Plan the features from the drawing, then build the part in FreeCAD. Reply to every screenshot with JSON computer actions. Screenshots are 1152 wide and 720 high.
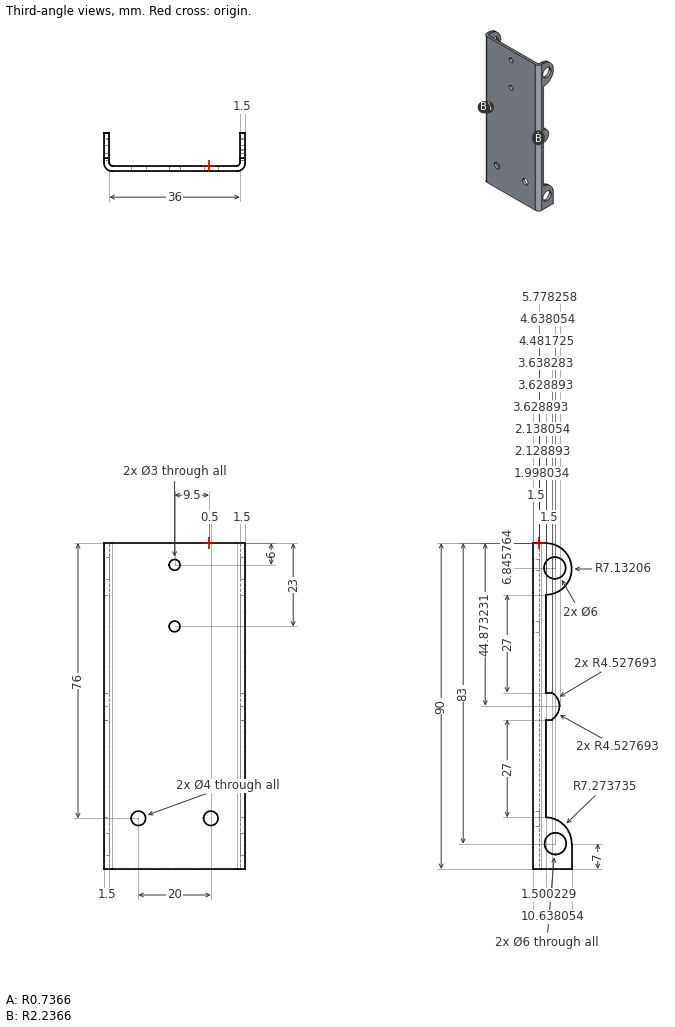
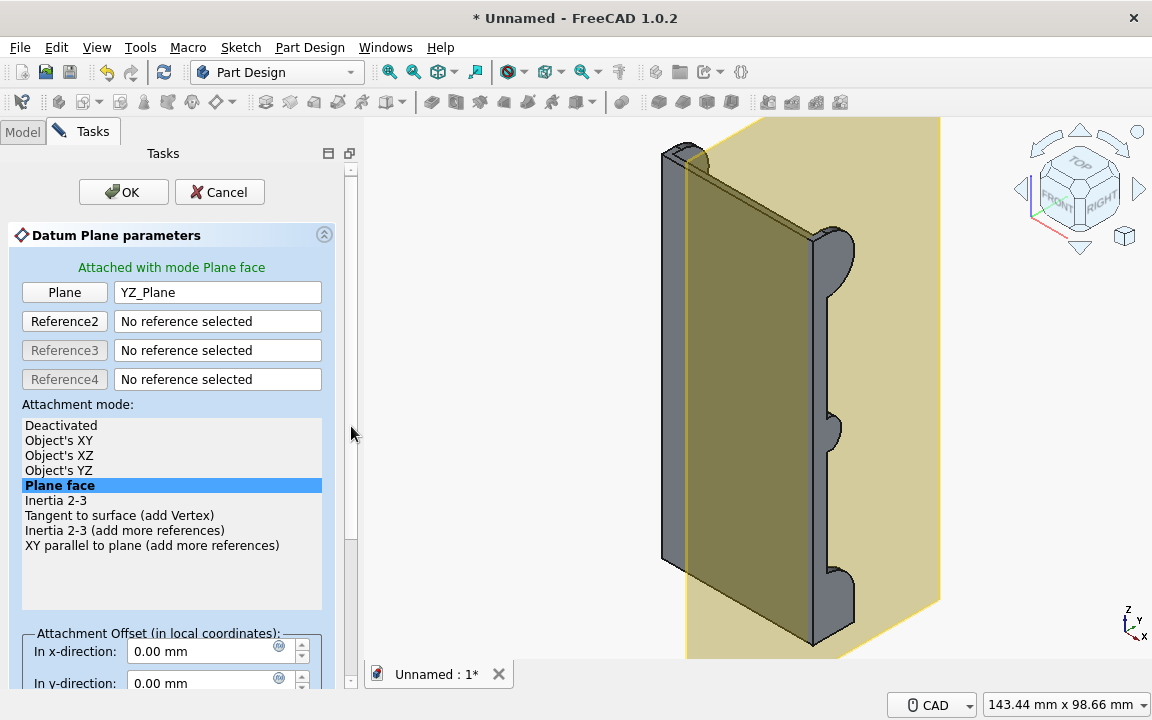
{"action": "left_click", "coordinate": [124, 192]}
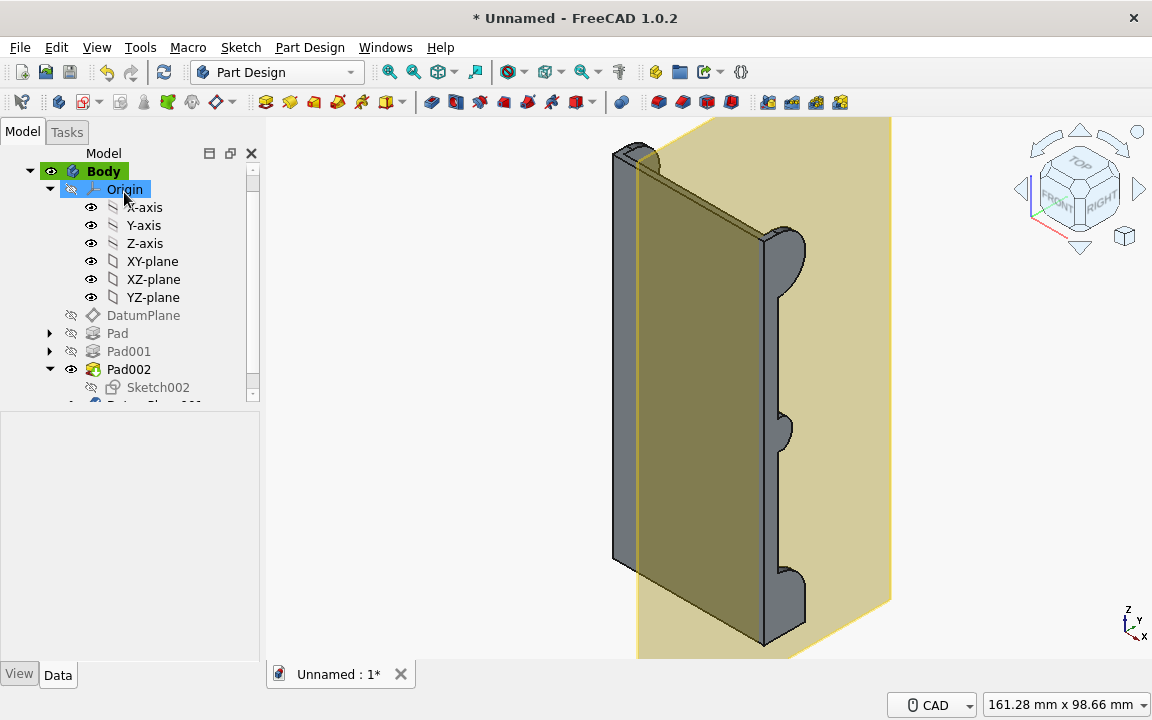
{"action": "scroll", "coordinate": [120, 275], "scroll_direction": "down", "scroll_amount": 3}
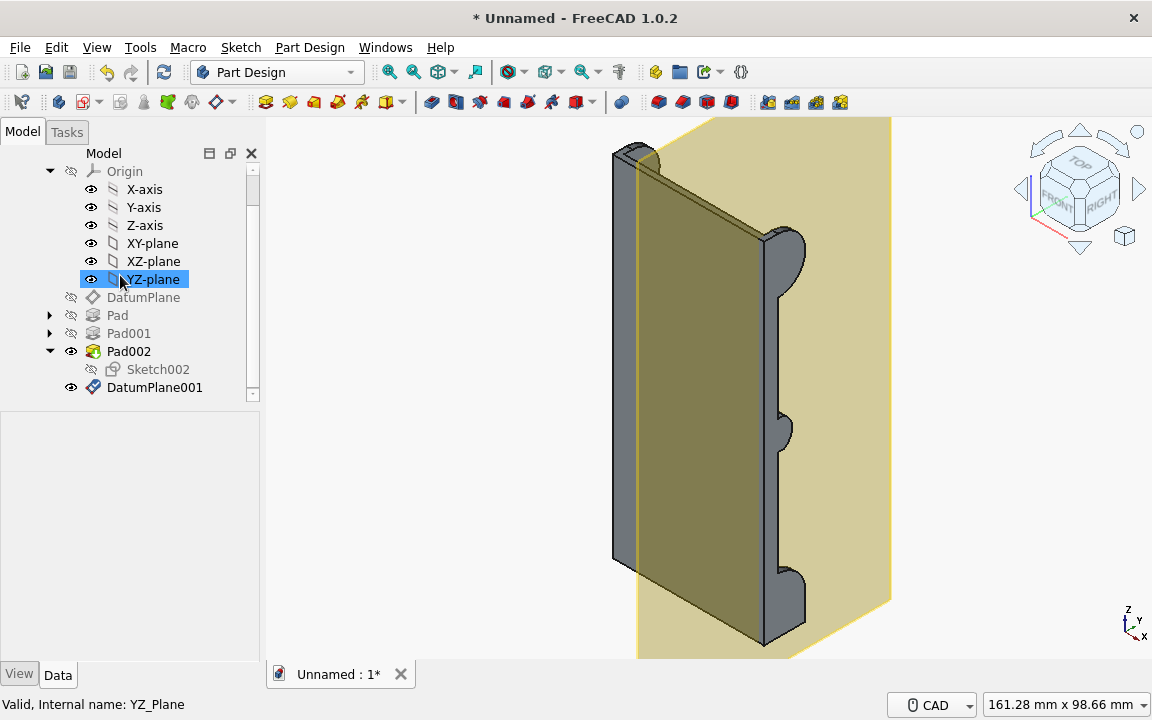
{"action": "left_click", "coordinate": [116, 387]}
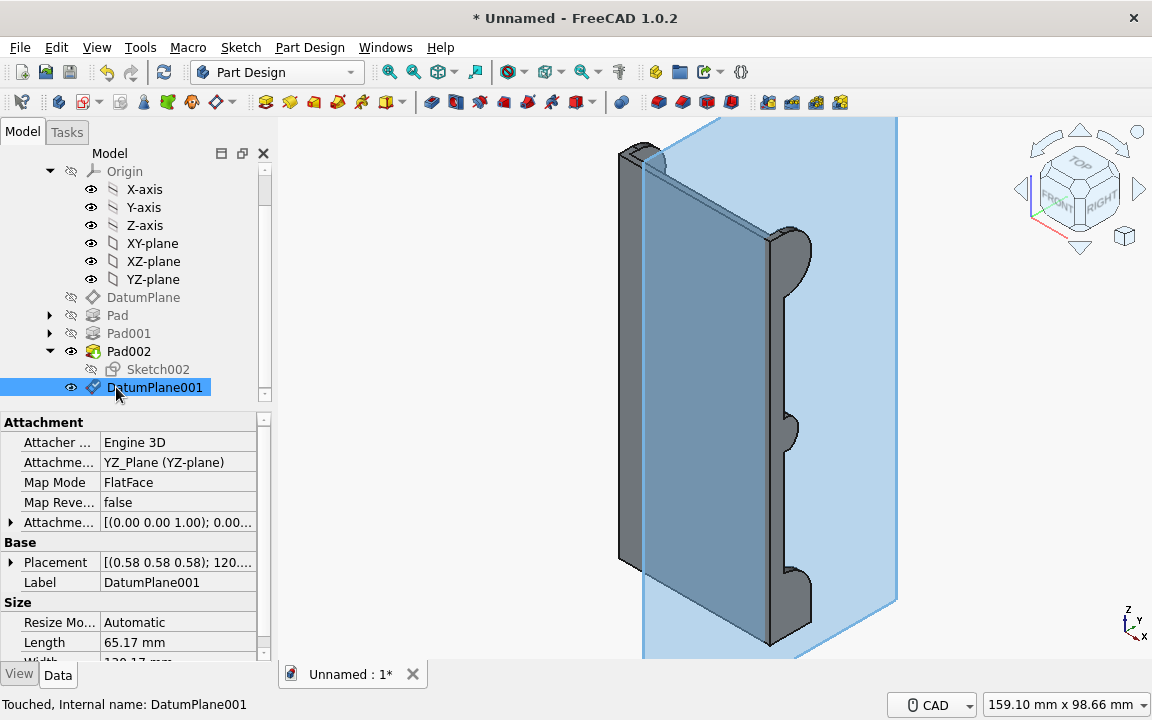
{"action": "left_click", "coordinate": [84, 102]}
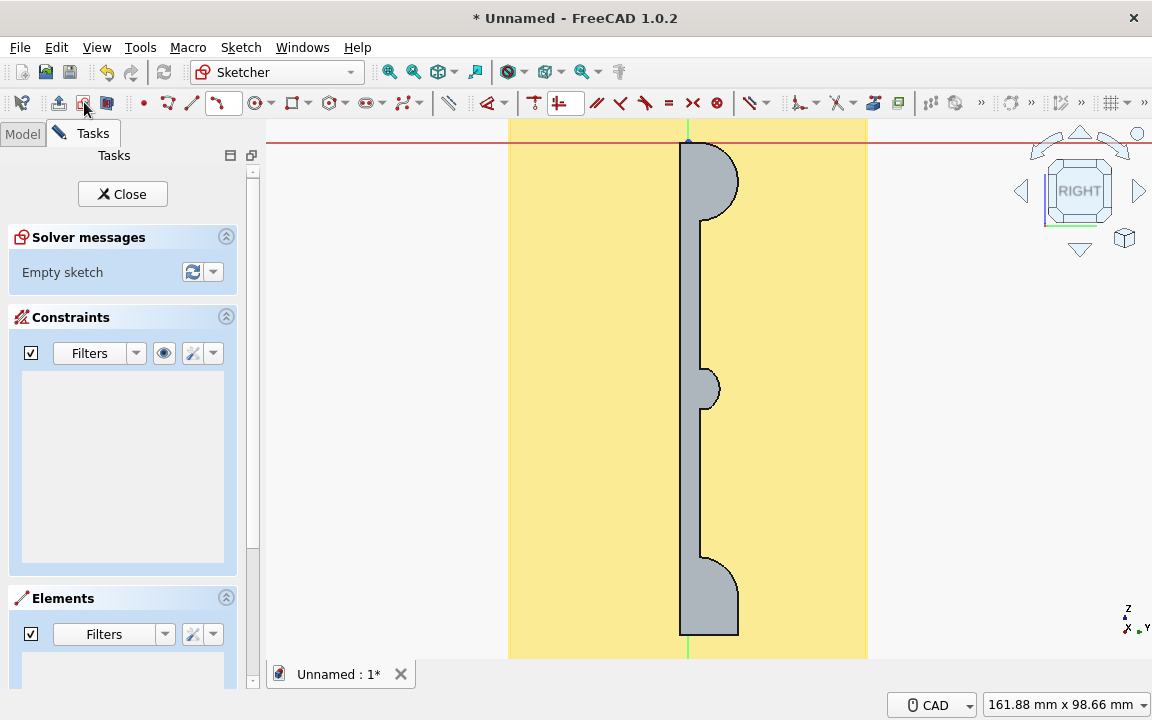
{"action": "key", "text": "q s"}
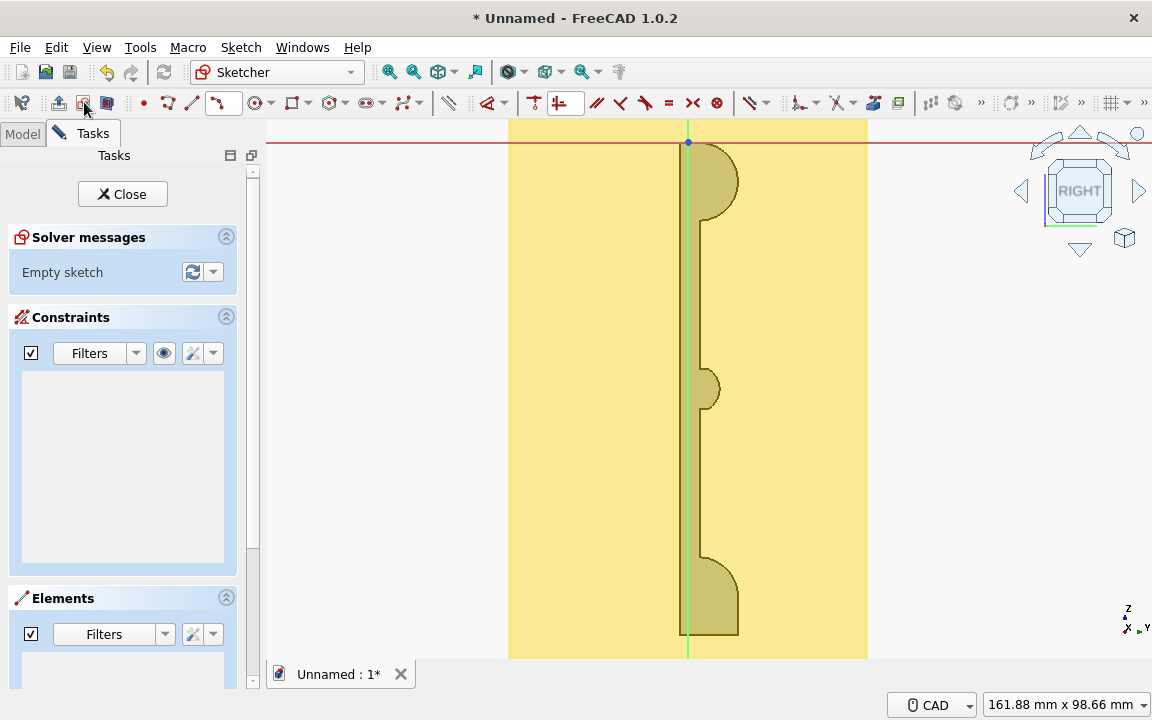
{"action": "scroll", "coordinate": [501, 411], "scroll_direction": "down", "scroll_amount": 2}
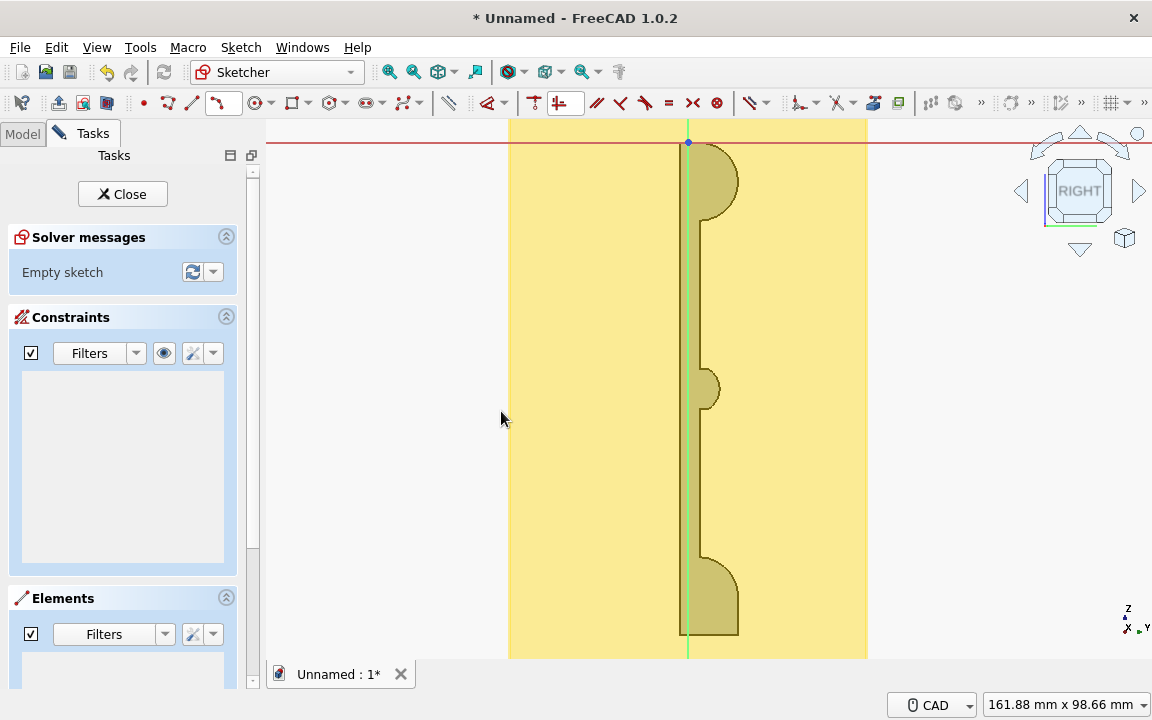
{"action": "left_click", "coordinate": [256, 104]}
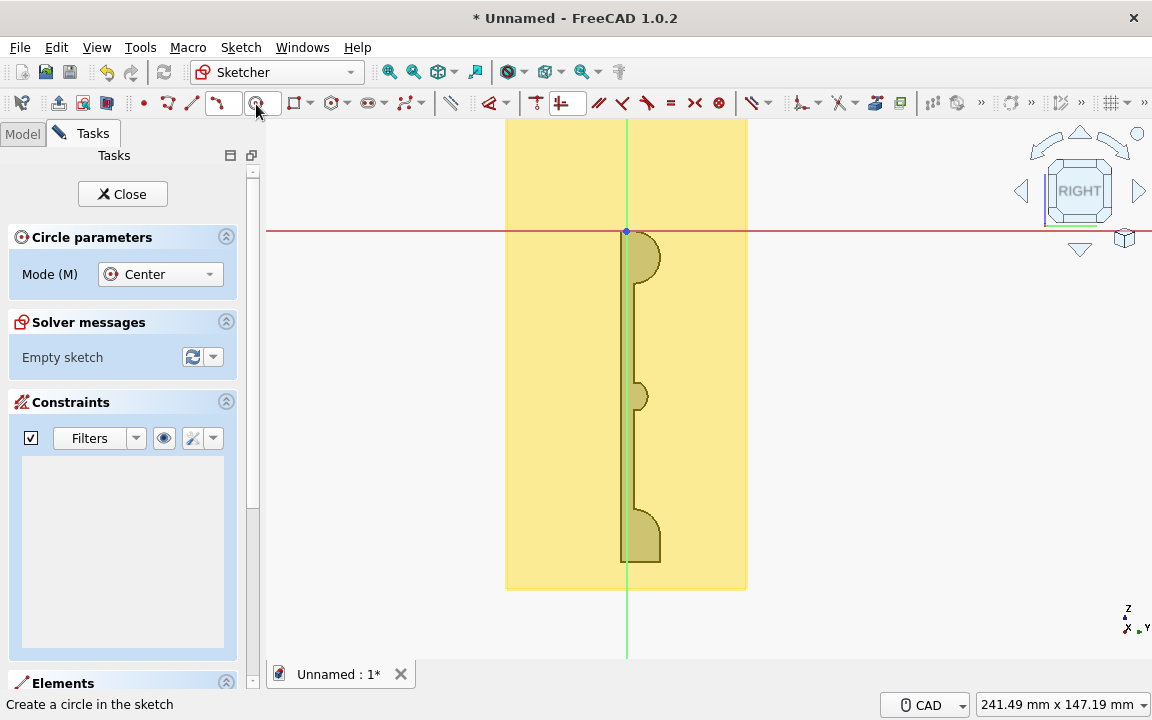
{"action": "scroll", "coordinate": [643, 256], "scroll_direction": "up", "scroll_amount": 4}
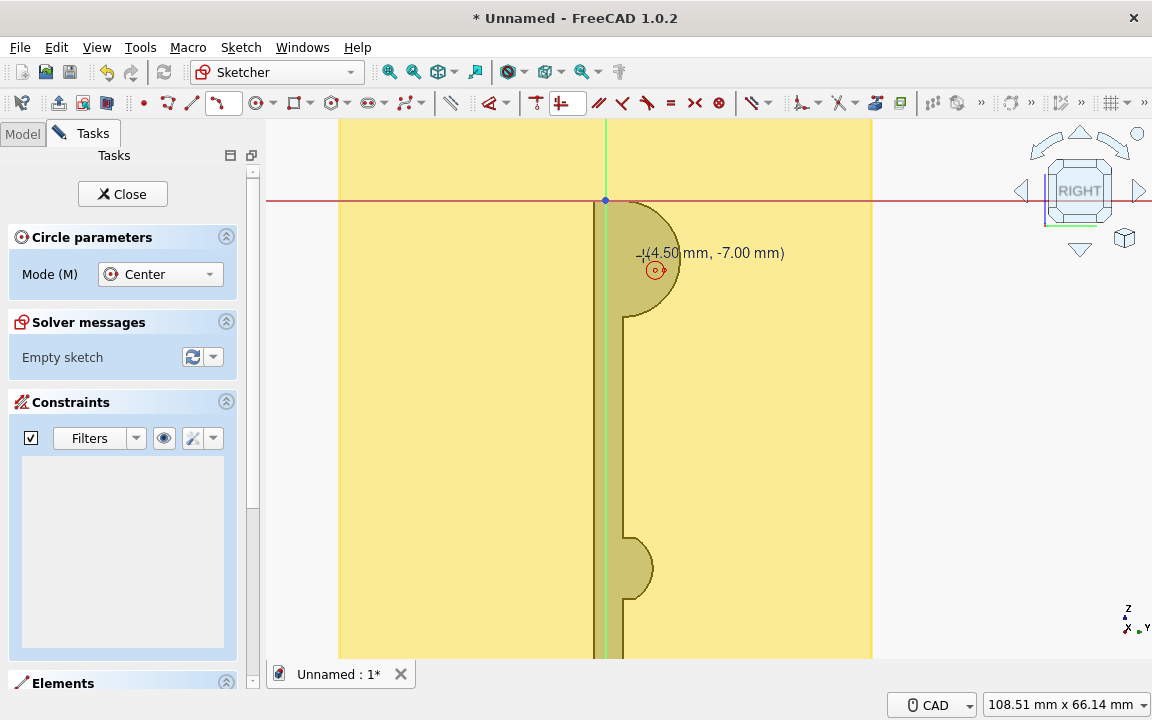
{"action": "left_click", "coordinate": [642, 257]}
{"action": "left_click", "coordinate": [660, 239]}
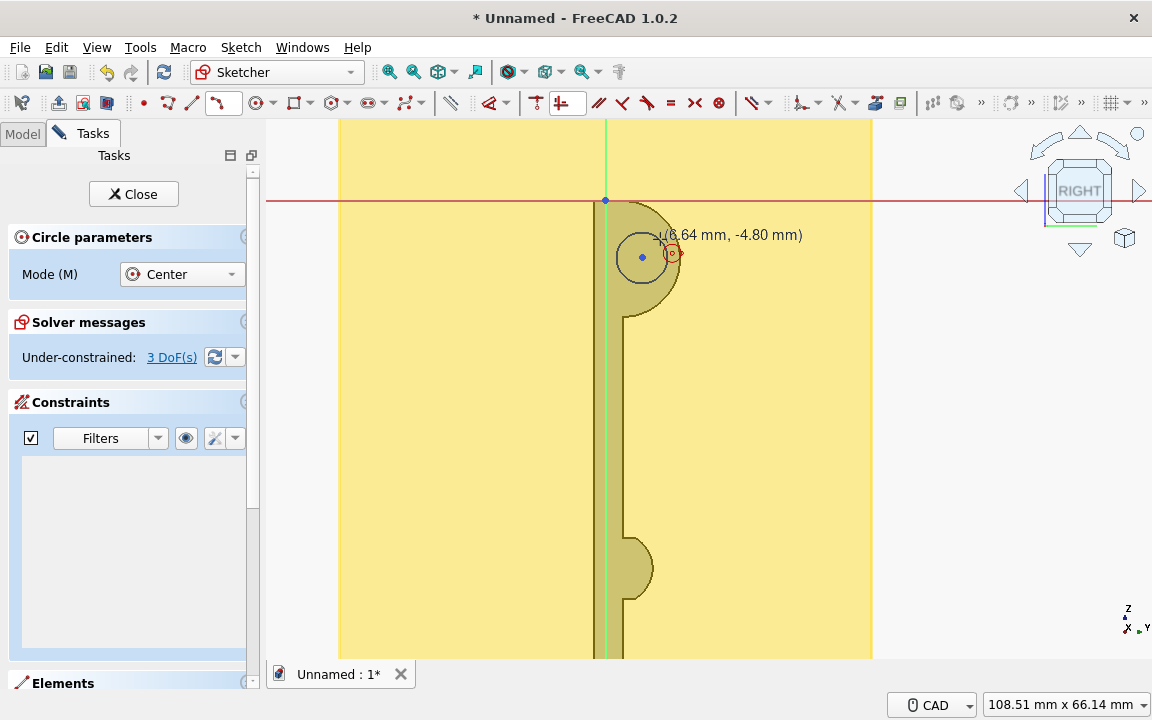
{"action": "scroll", "coordinate": [643, 256], "scroll_direction": "down", "scroll_amount": 4}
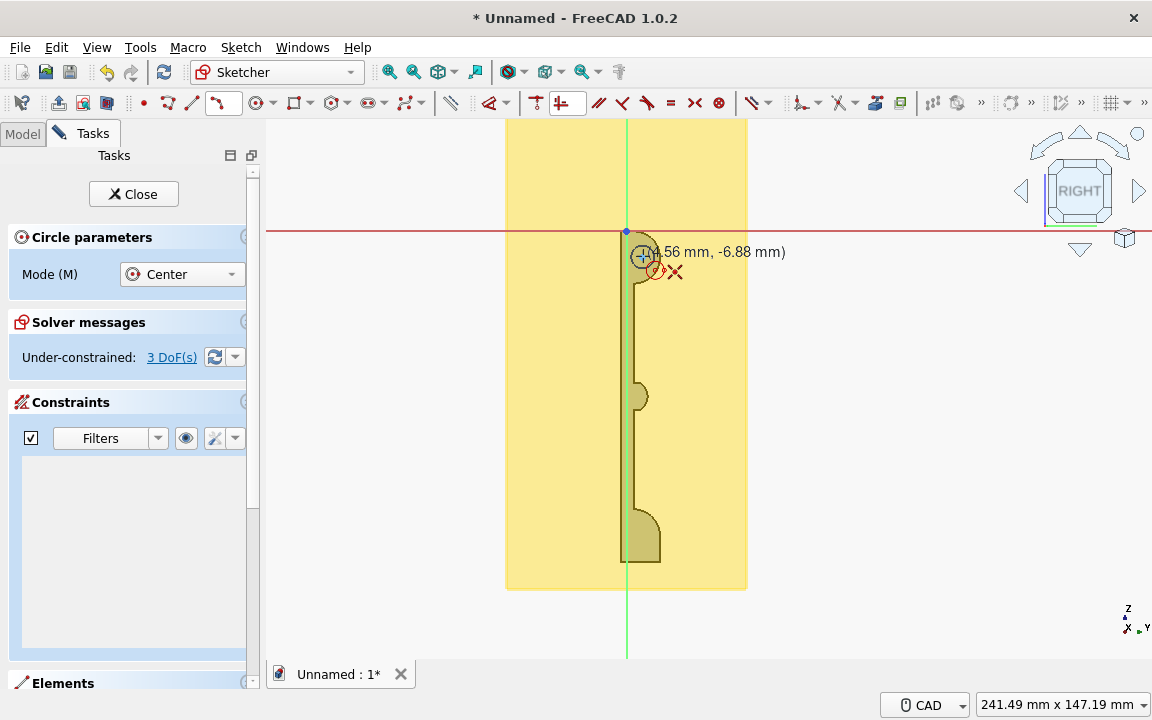
{"action": "scroll", "coordinate": [644, 536], "scroll_direction": "up", "scroll_amount": 4}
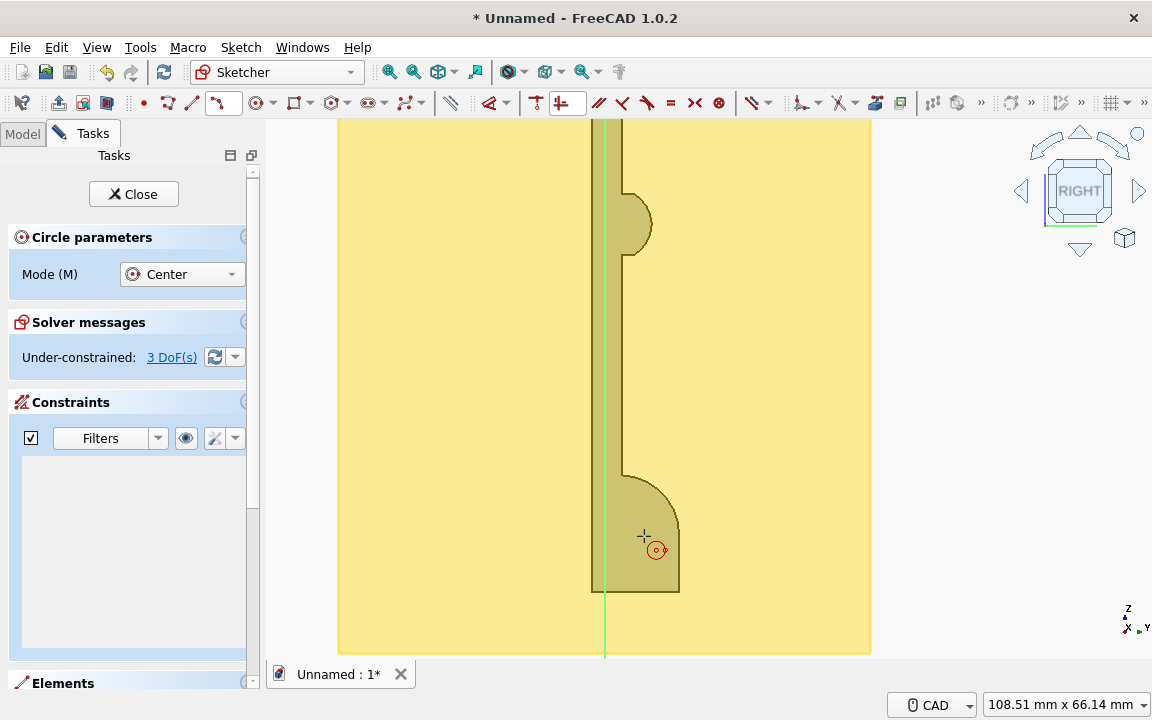
{"action": "left_click", "coordinate": [642, 535]}
{"action": "left_click", "coordinate": [660, 517]}
{"action": "key", "text": "Escape"}